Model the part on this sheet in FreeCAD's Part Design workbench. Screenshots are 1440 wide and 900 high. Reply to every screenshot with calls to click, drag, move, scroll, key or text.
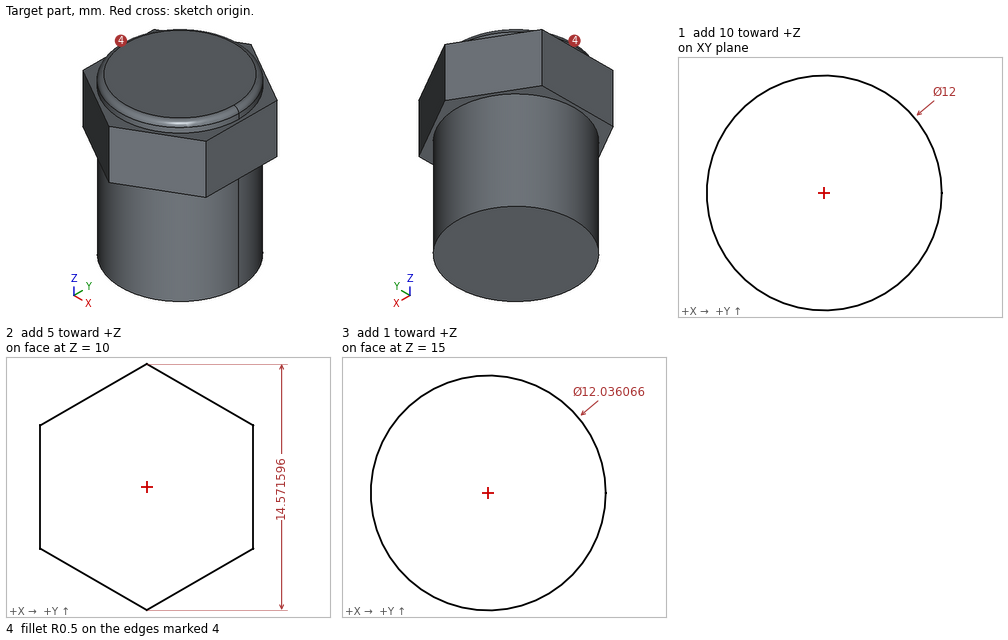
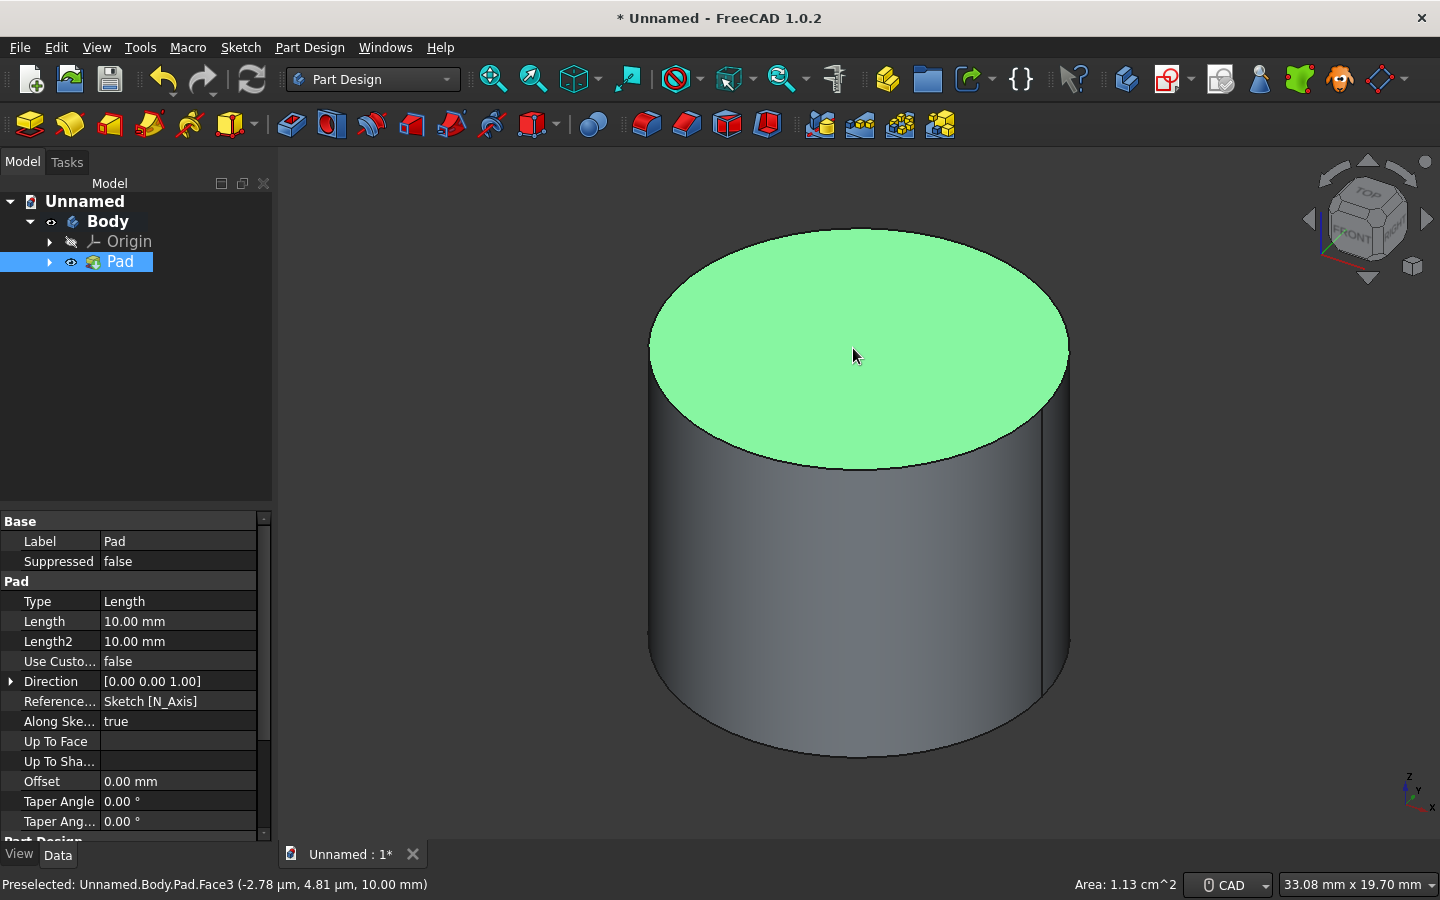
click(1168, 80)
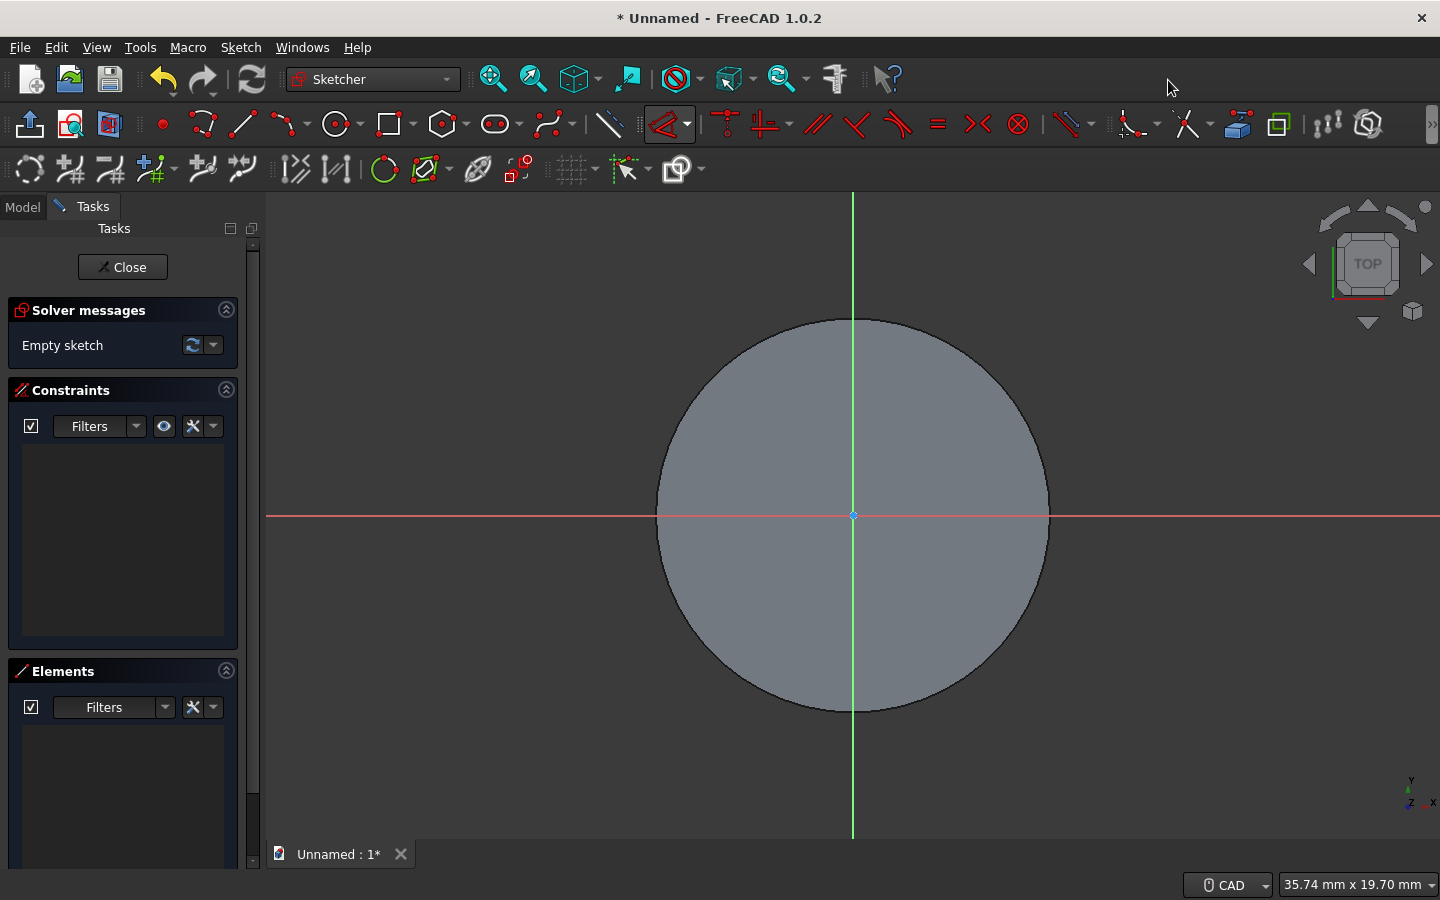
click(442, 124)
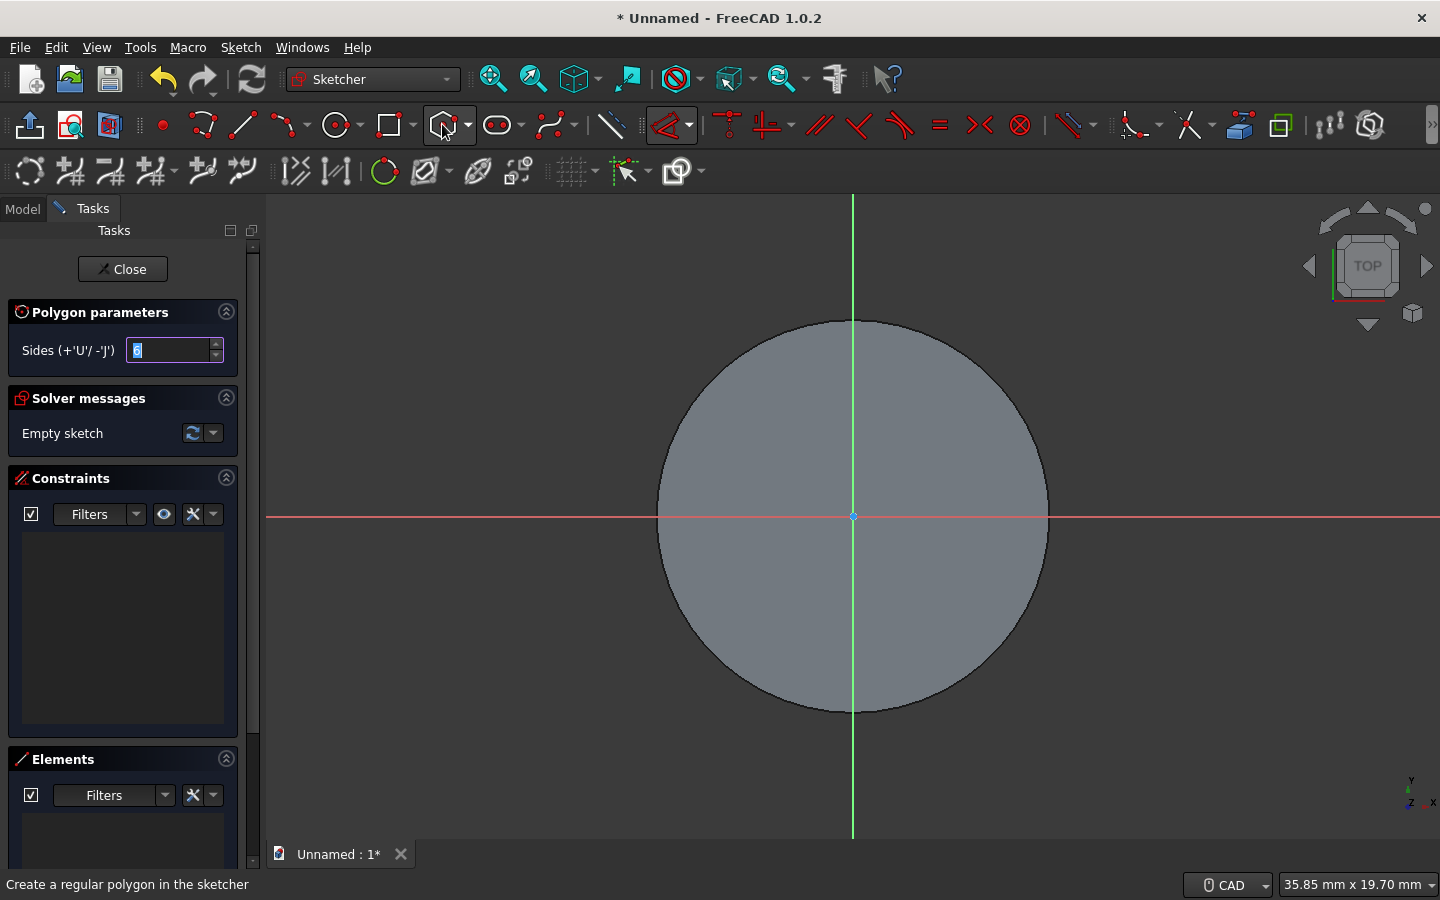
click(853, 516)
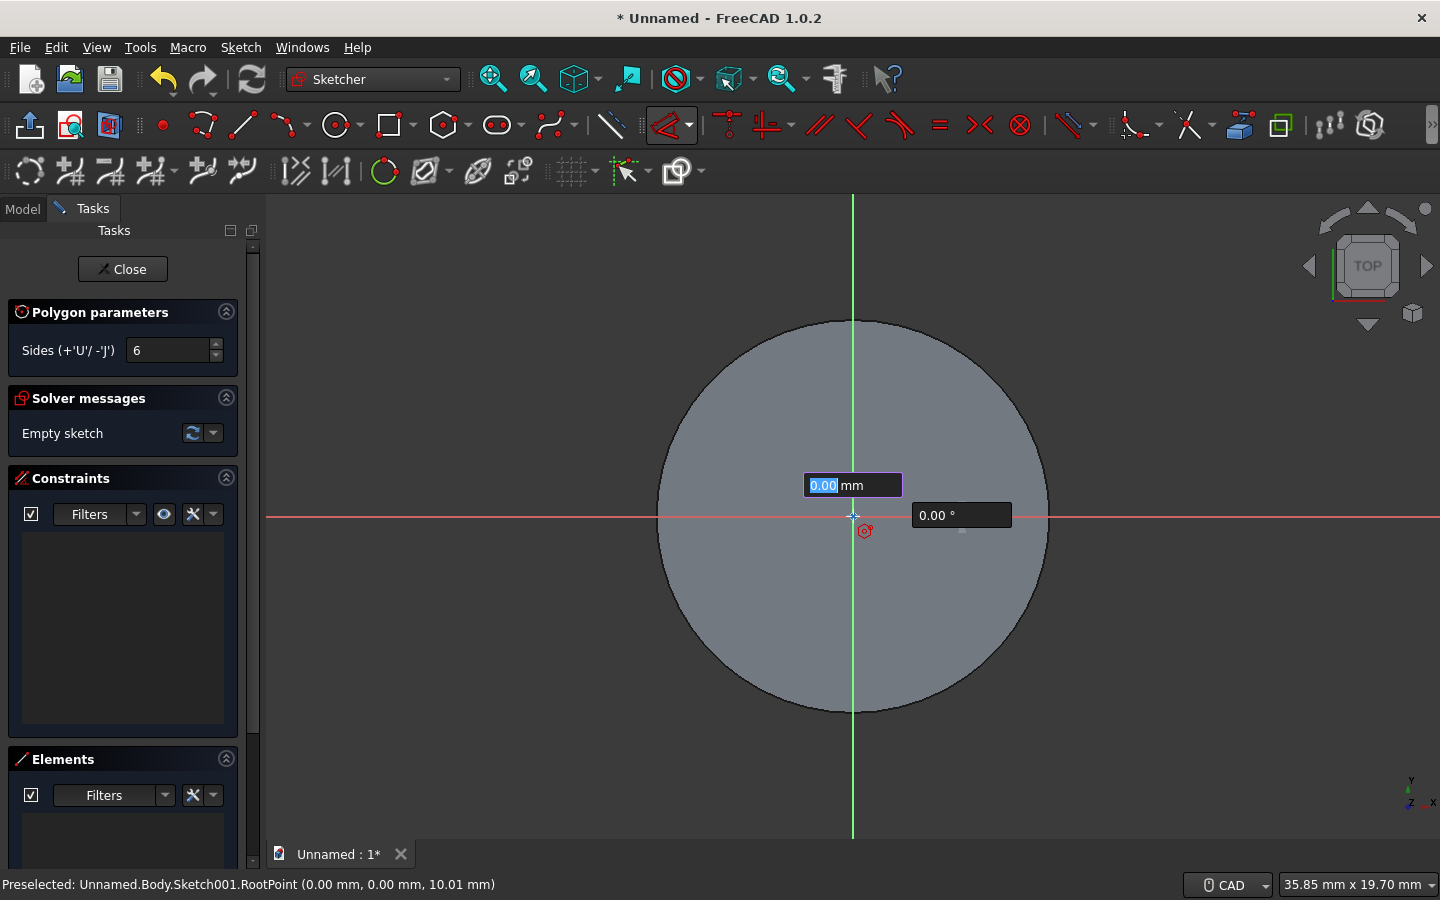
click(853, 278)
key(Escape)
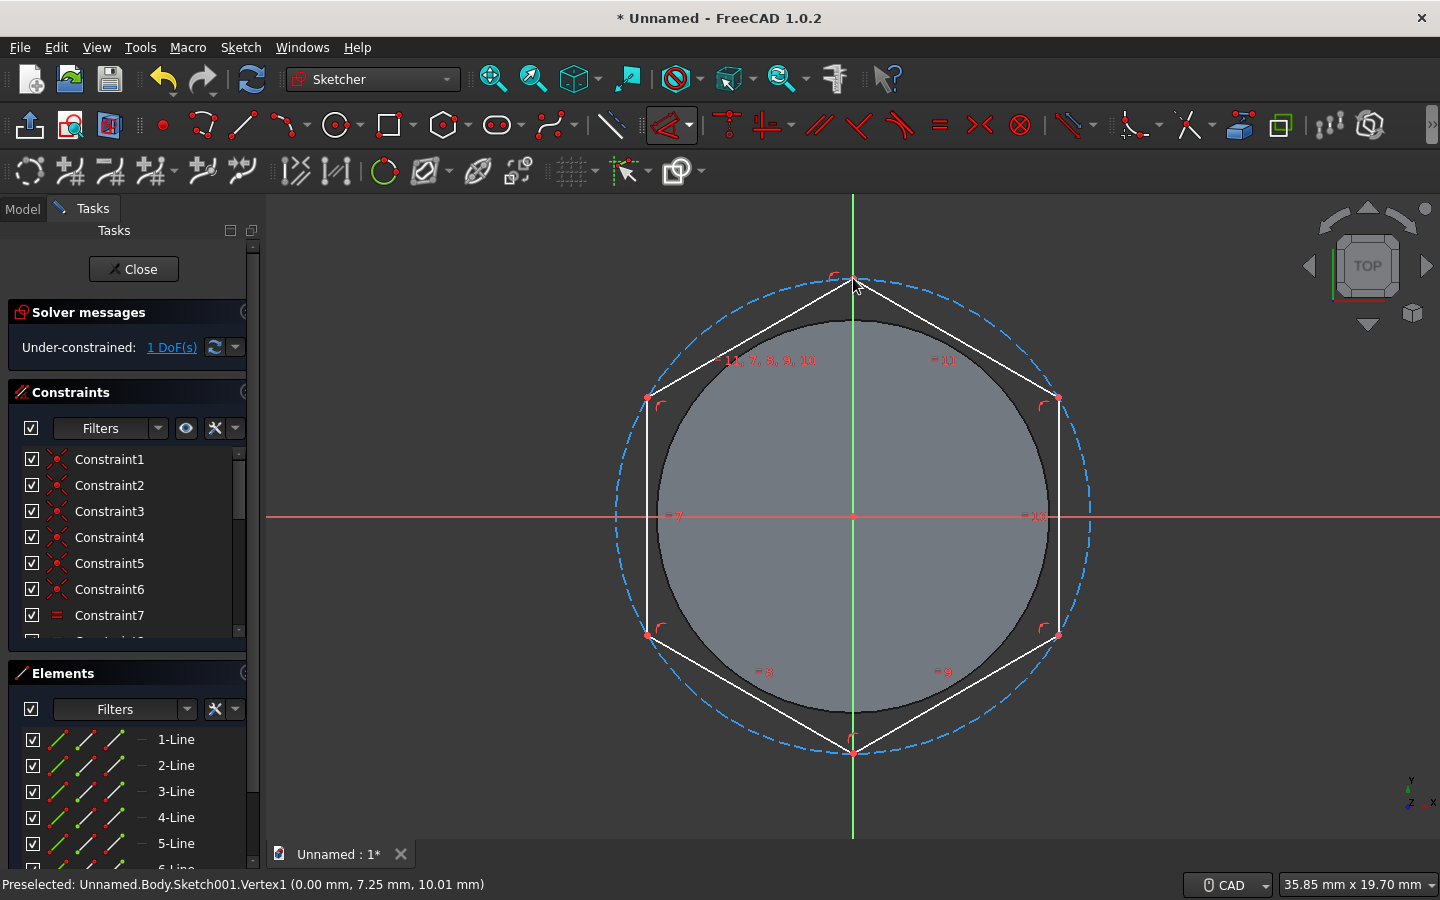
click(853, 754)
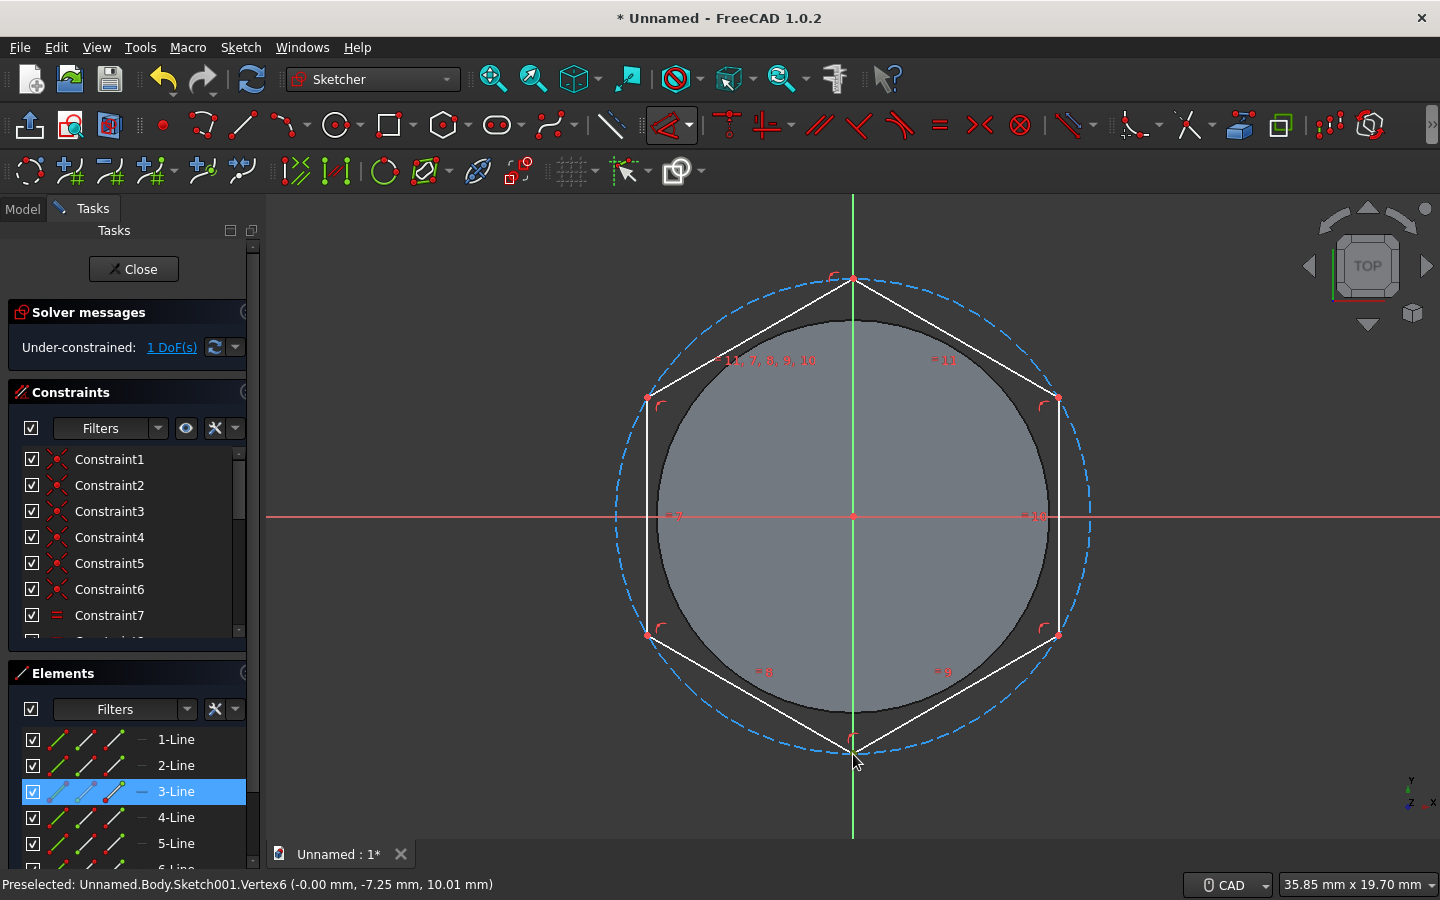
click(853, 279)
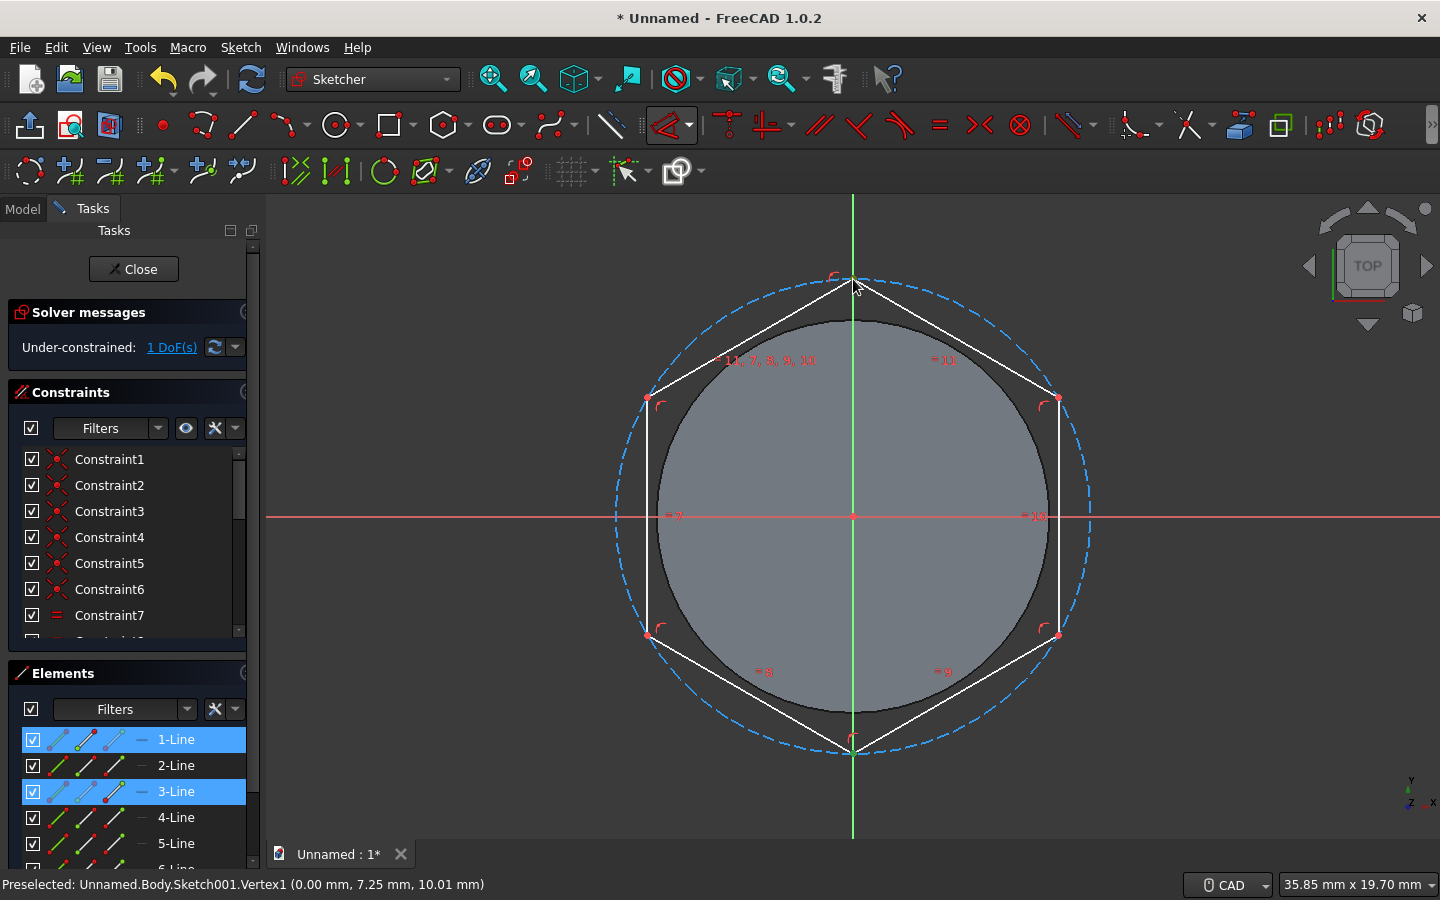
key(i)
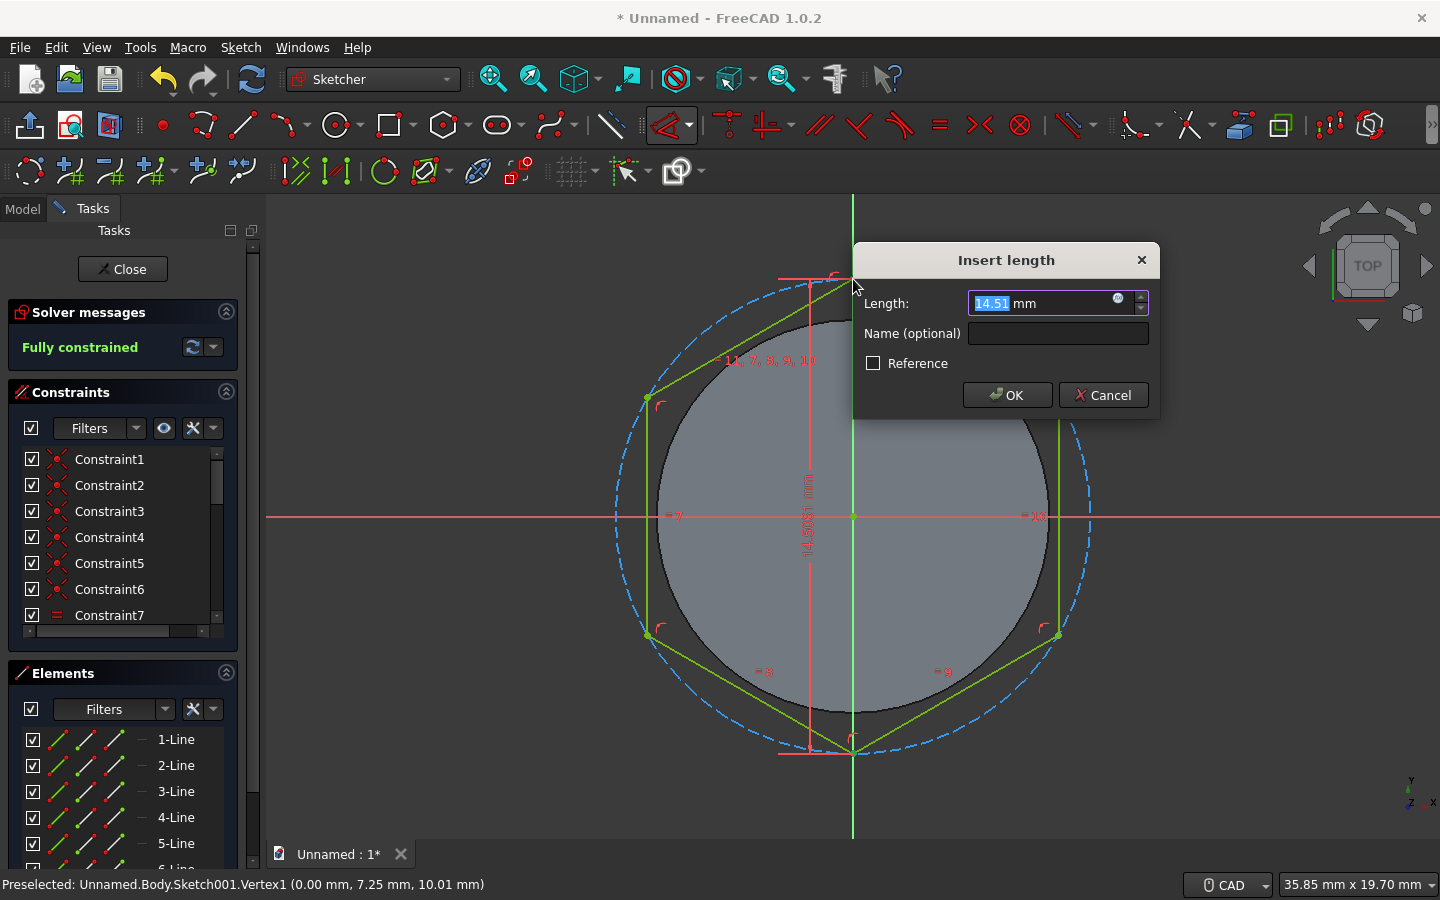
text(14.571596)
key(Return)